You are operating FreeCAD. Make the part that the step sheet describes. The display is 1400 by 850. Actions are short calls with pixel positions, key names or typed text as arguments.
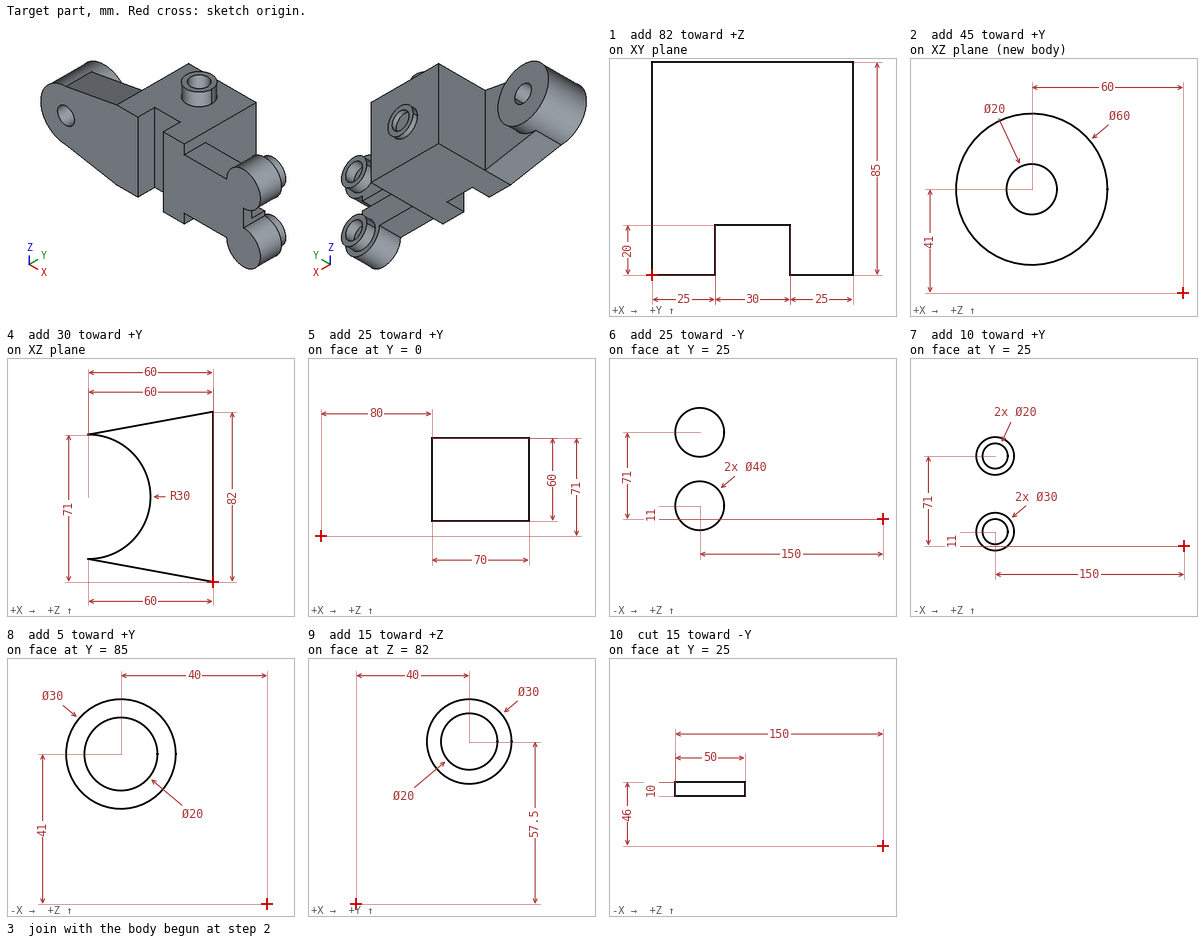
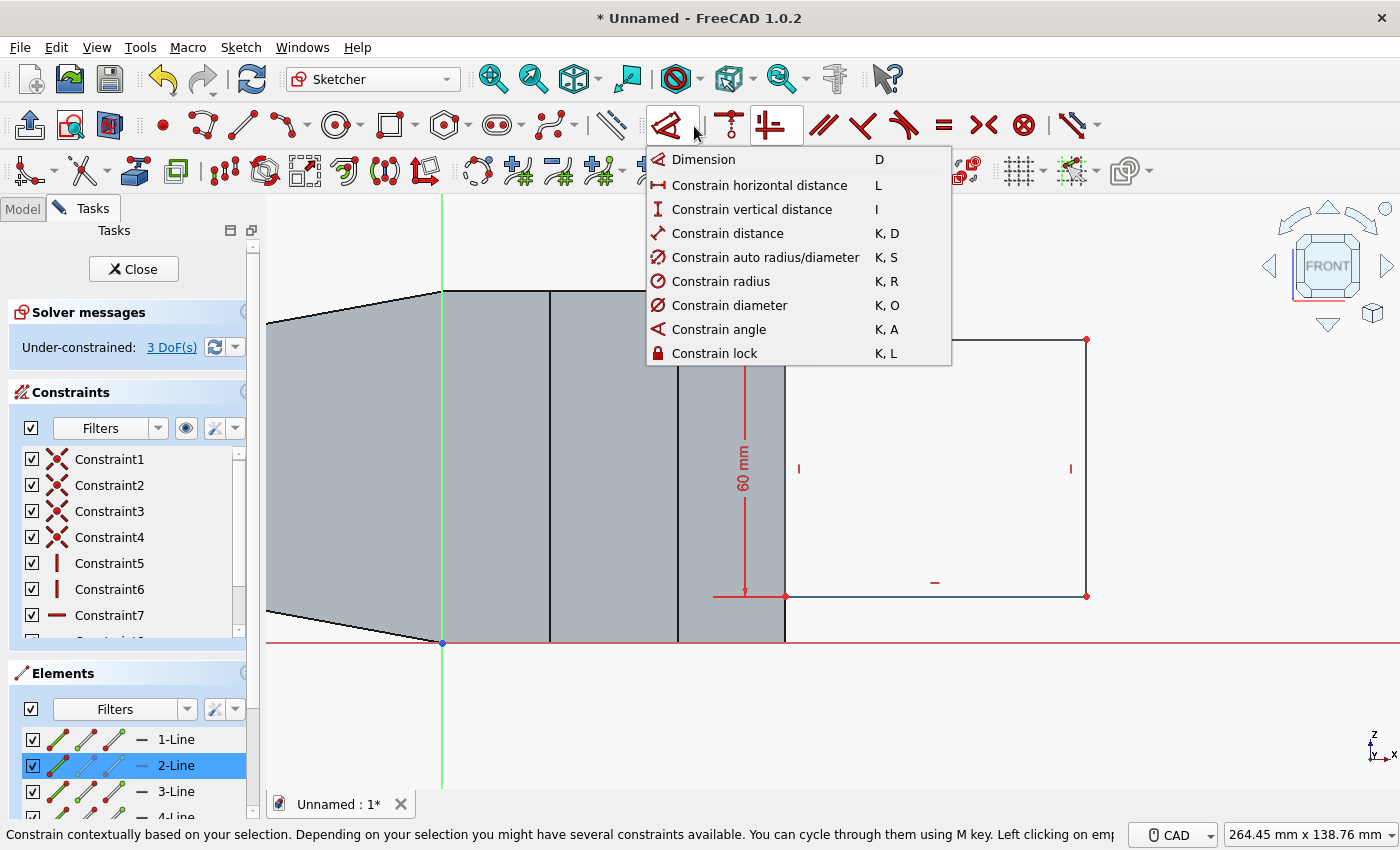
click(799, 185)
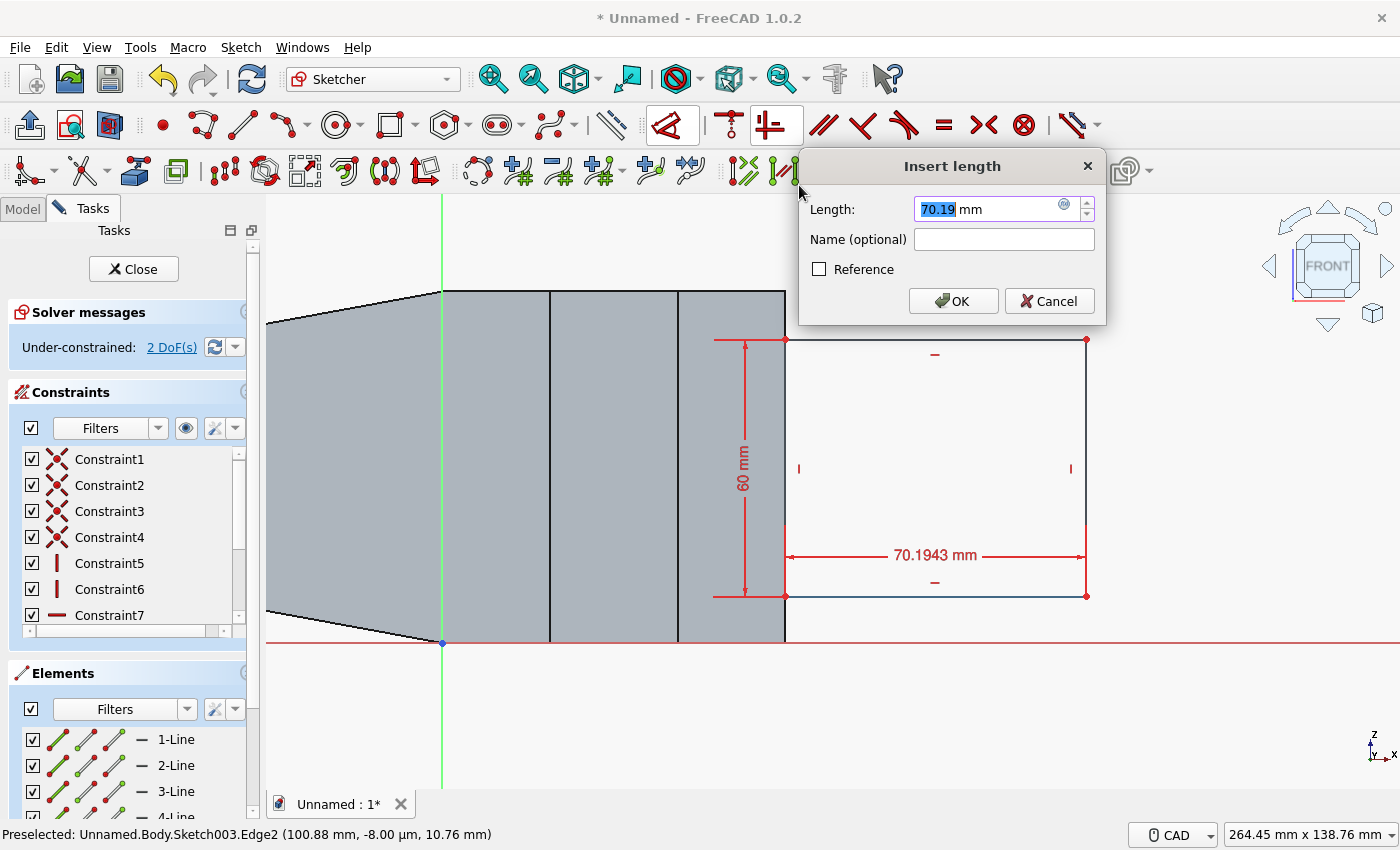
text(70)
key(Return)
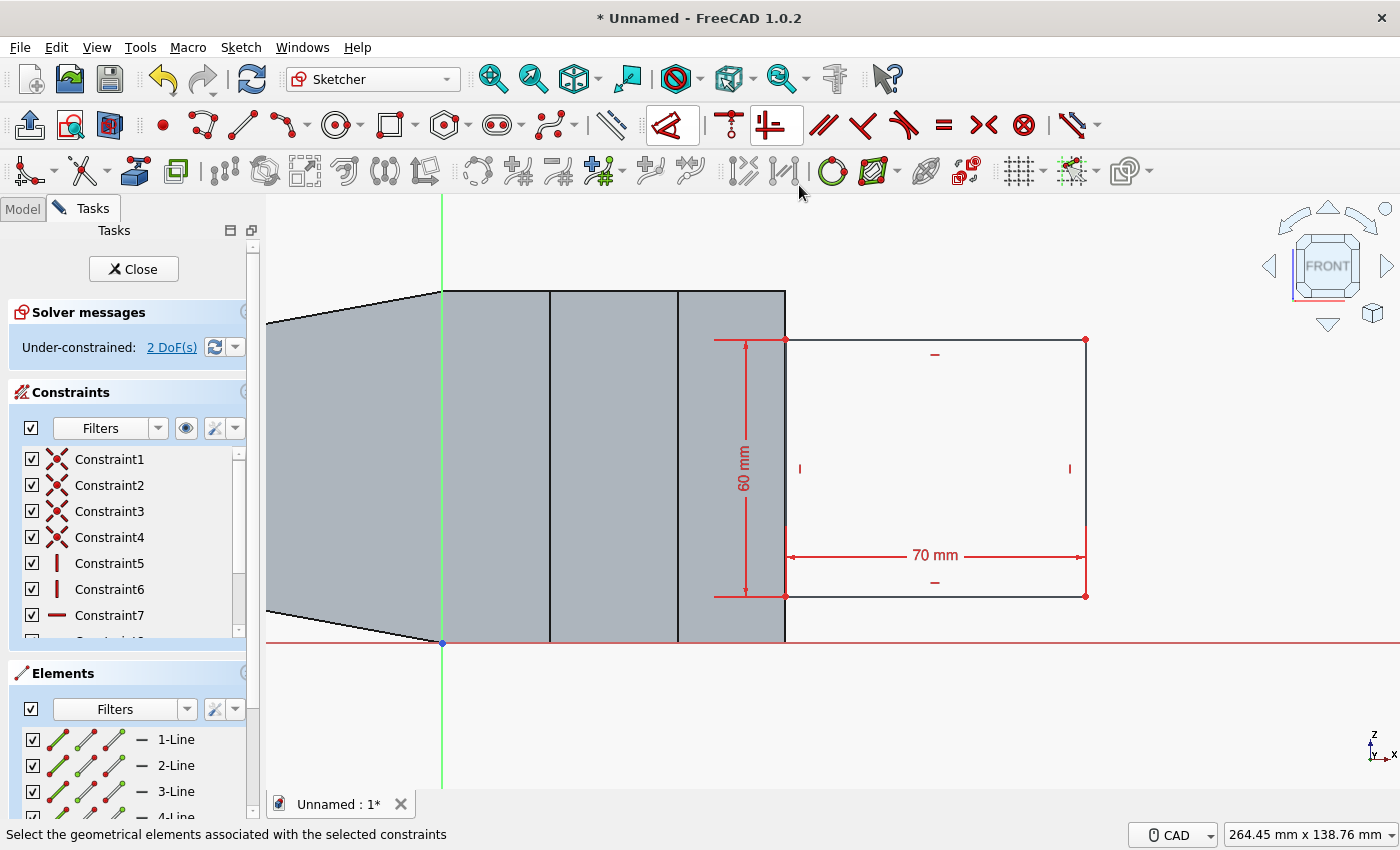
click(786, 340)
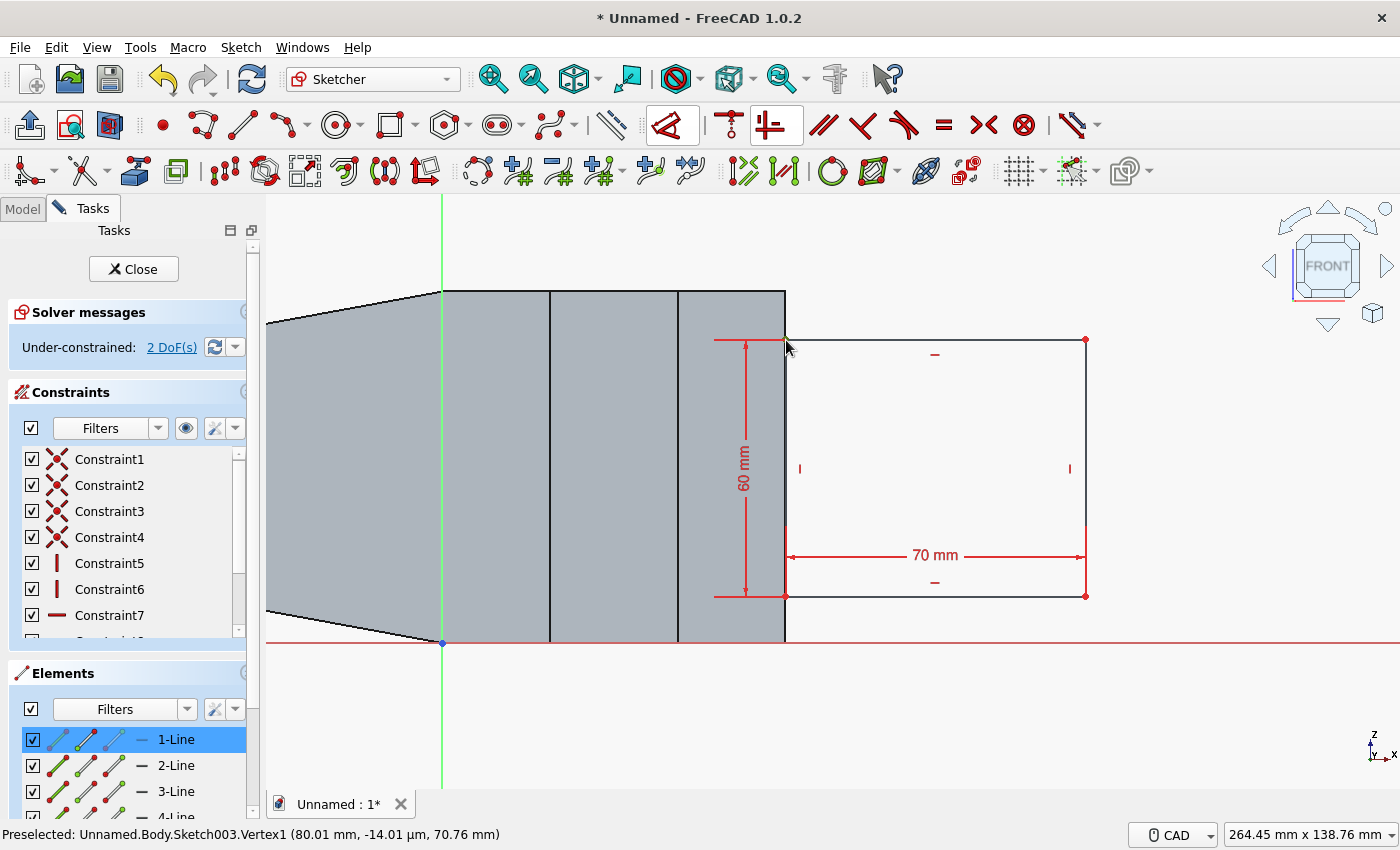
click(694, 126)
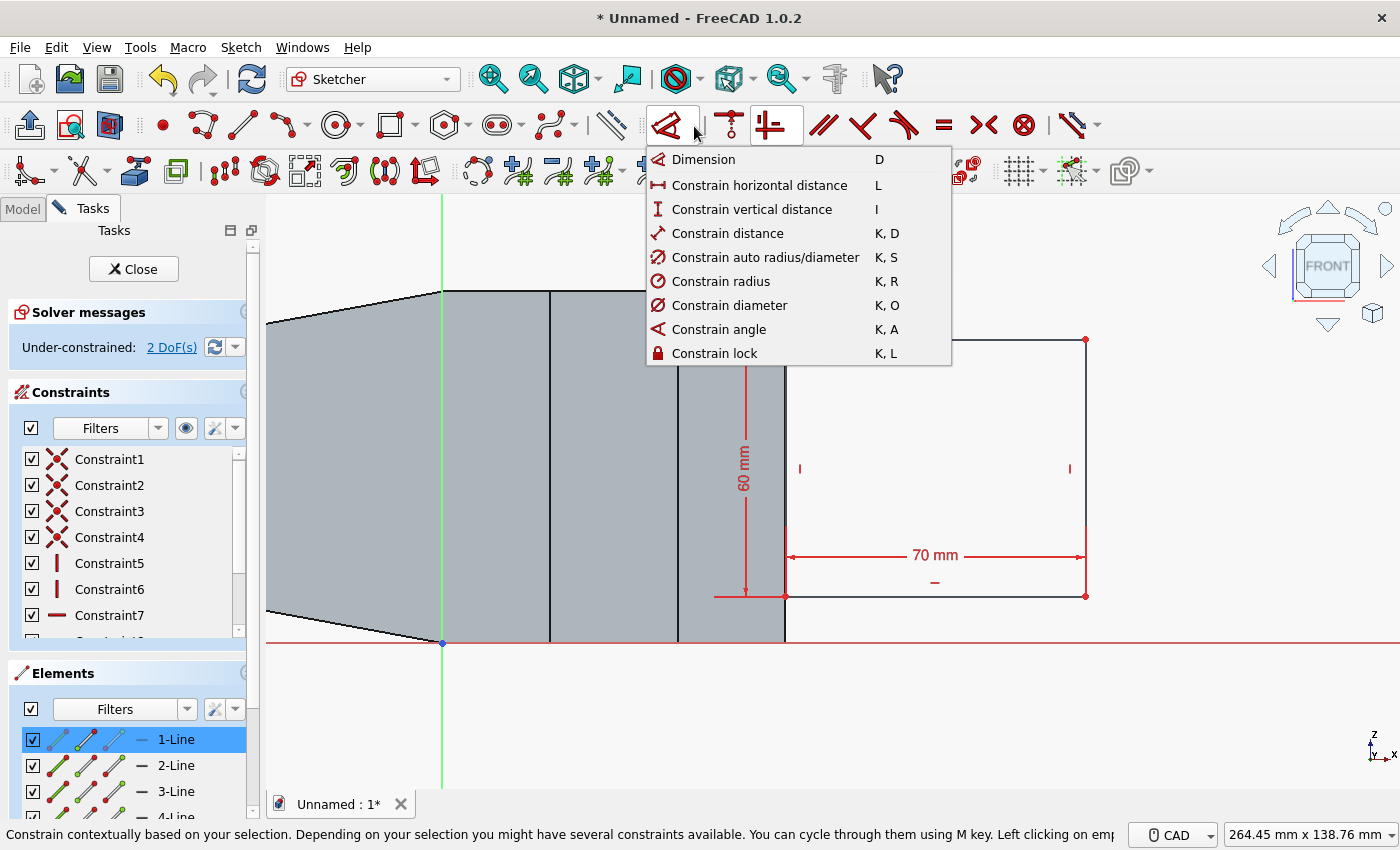
click(799, 185)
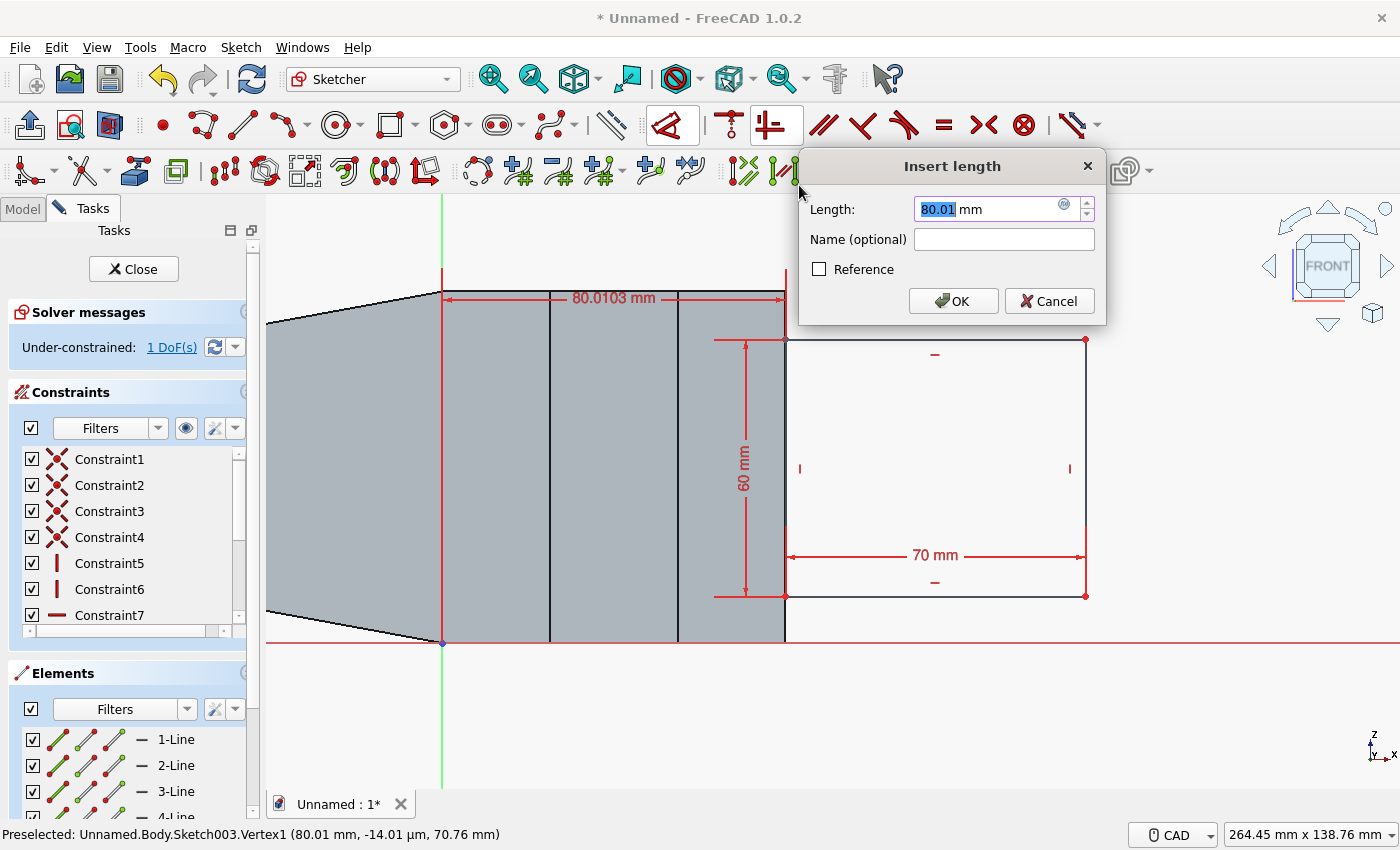
text(80)
key(Return)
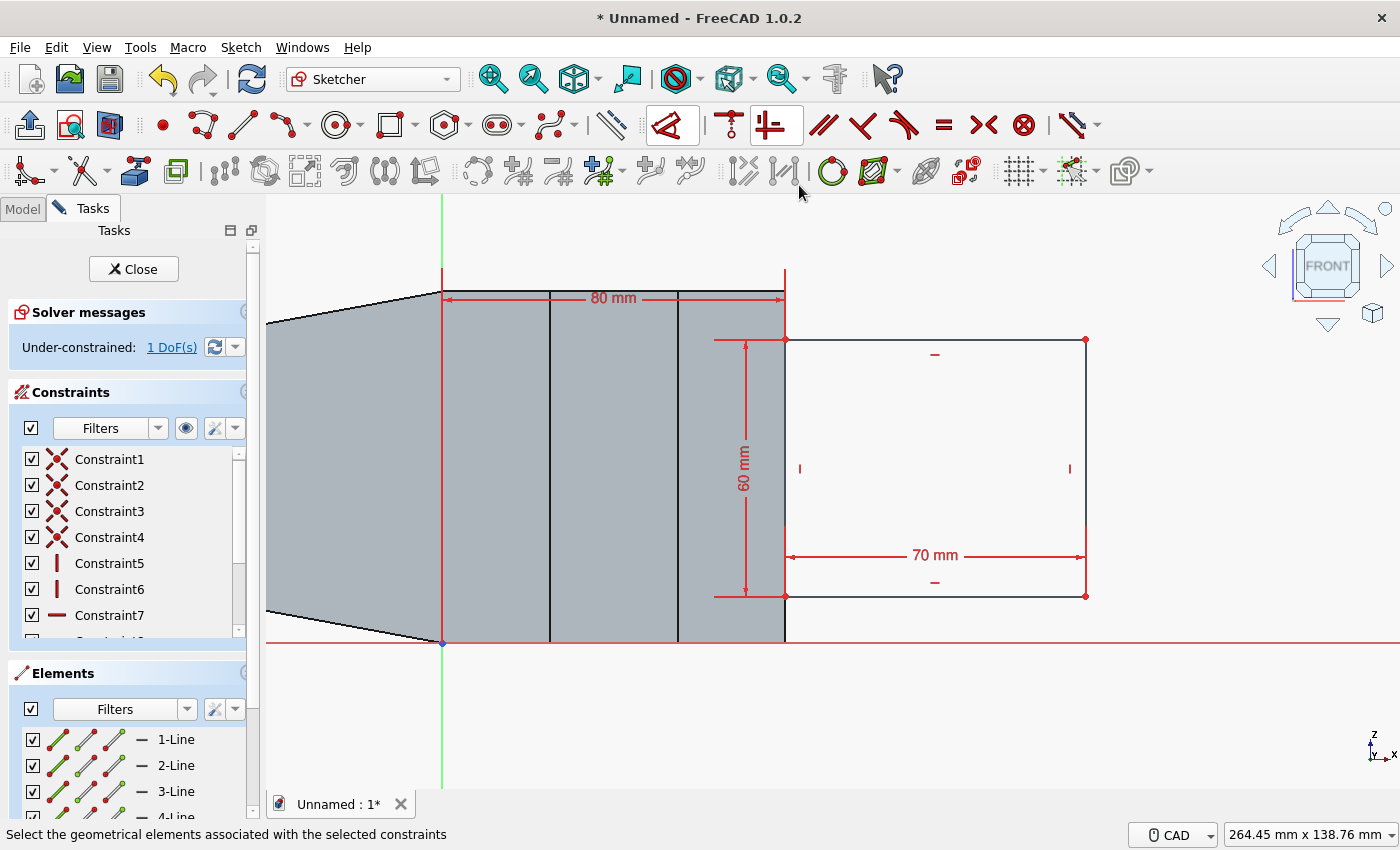
click(785, 340)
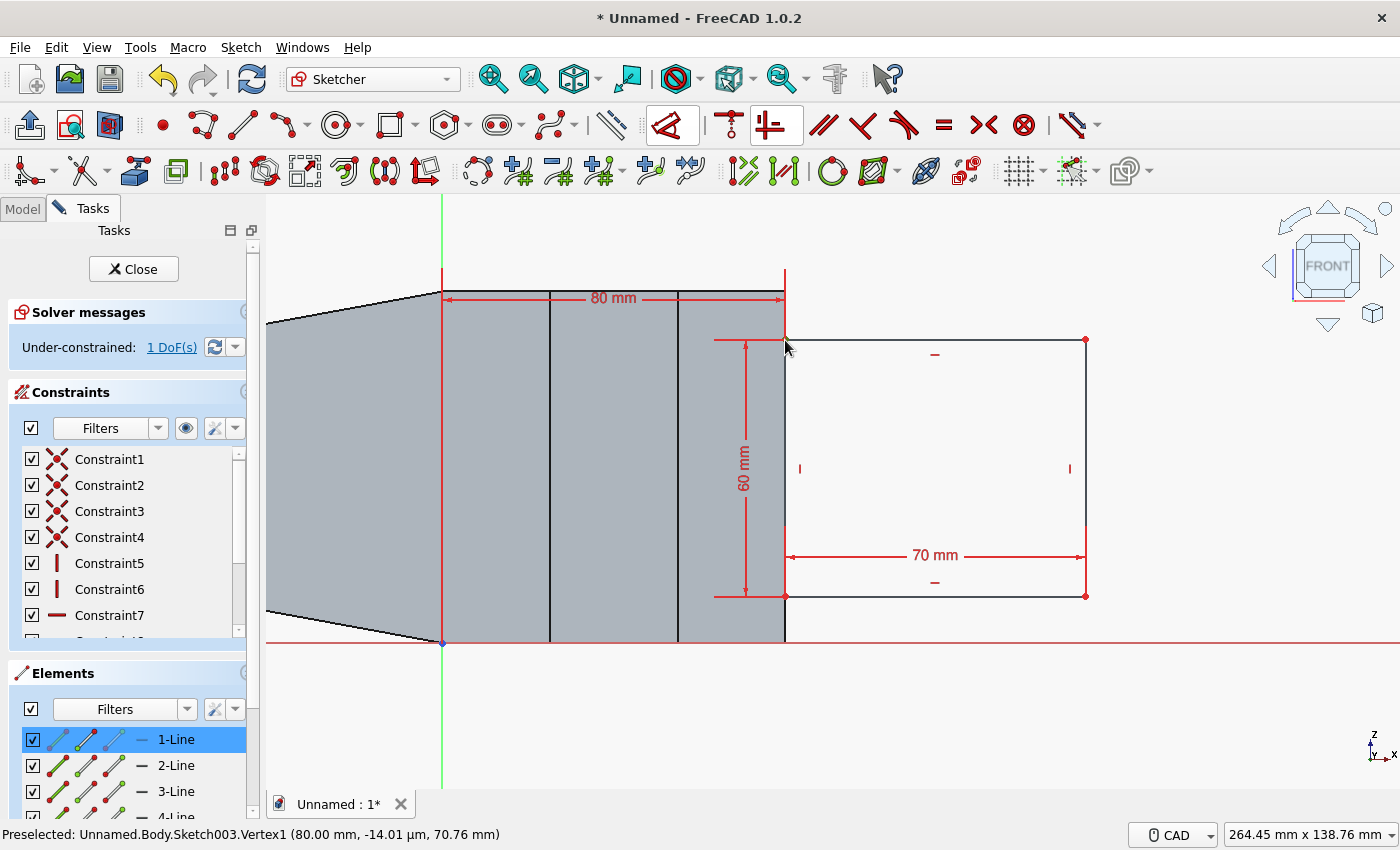
key(i)